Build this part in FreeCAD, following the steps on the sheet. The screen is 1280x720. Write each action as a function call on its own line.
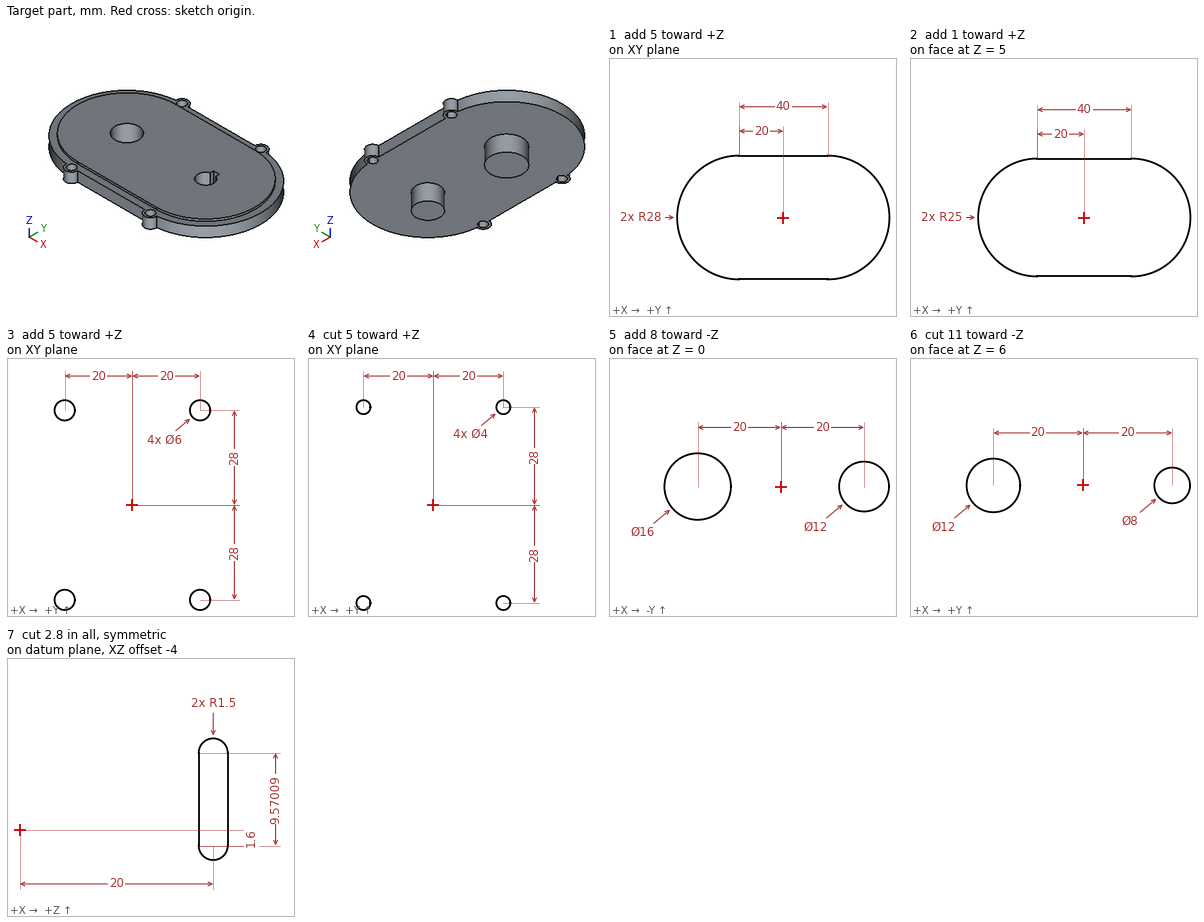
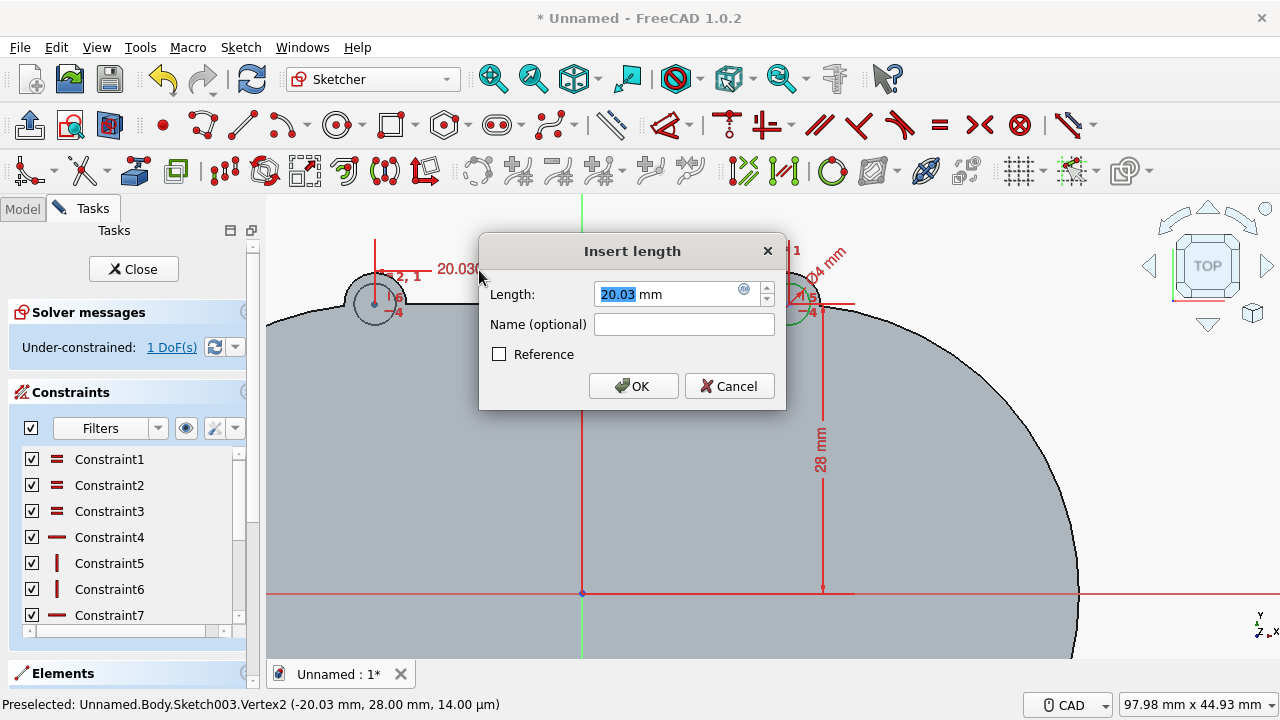
text(20)
key(Return)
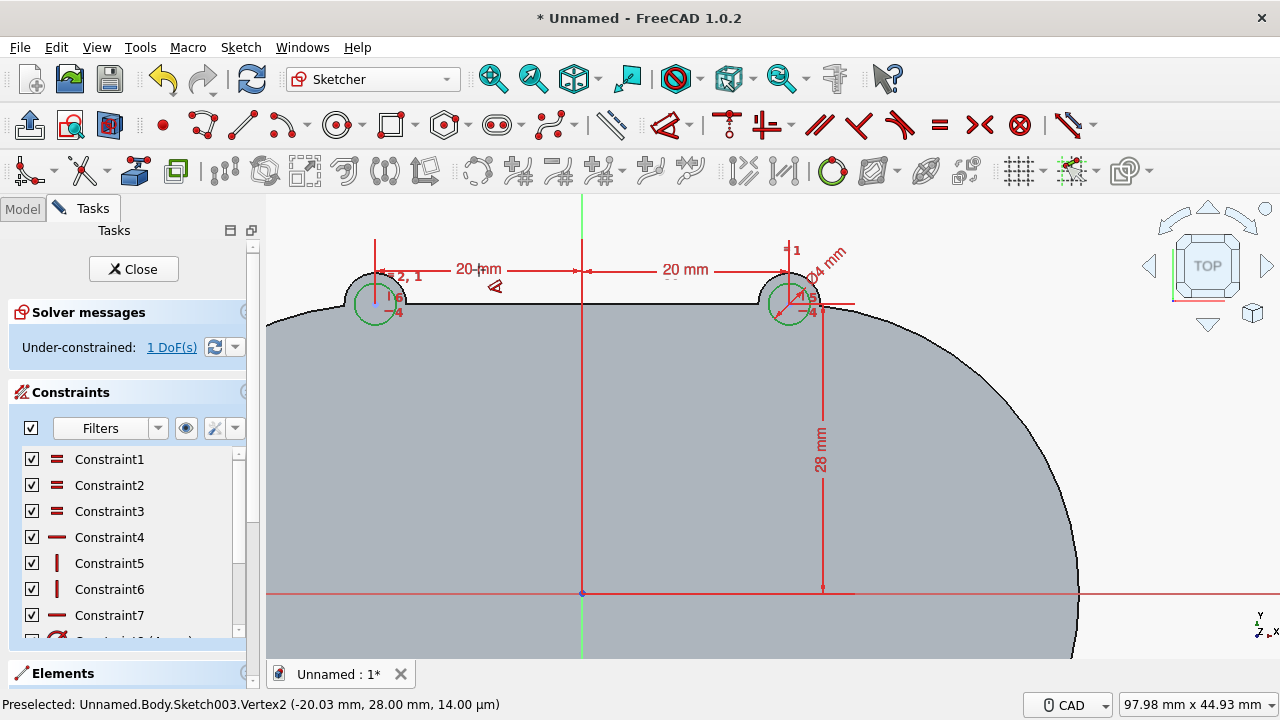
scroll(804, 290, down, 4)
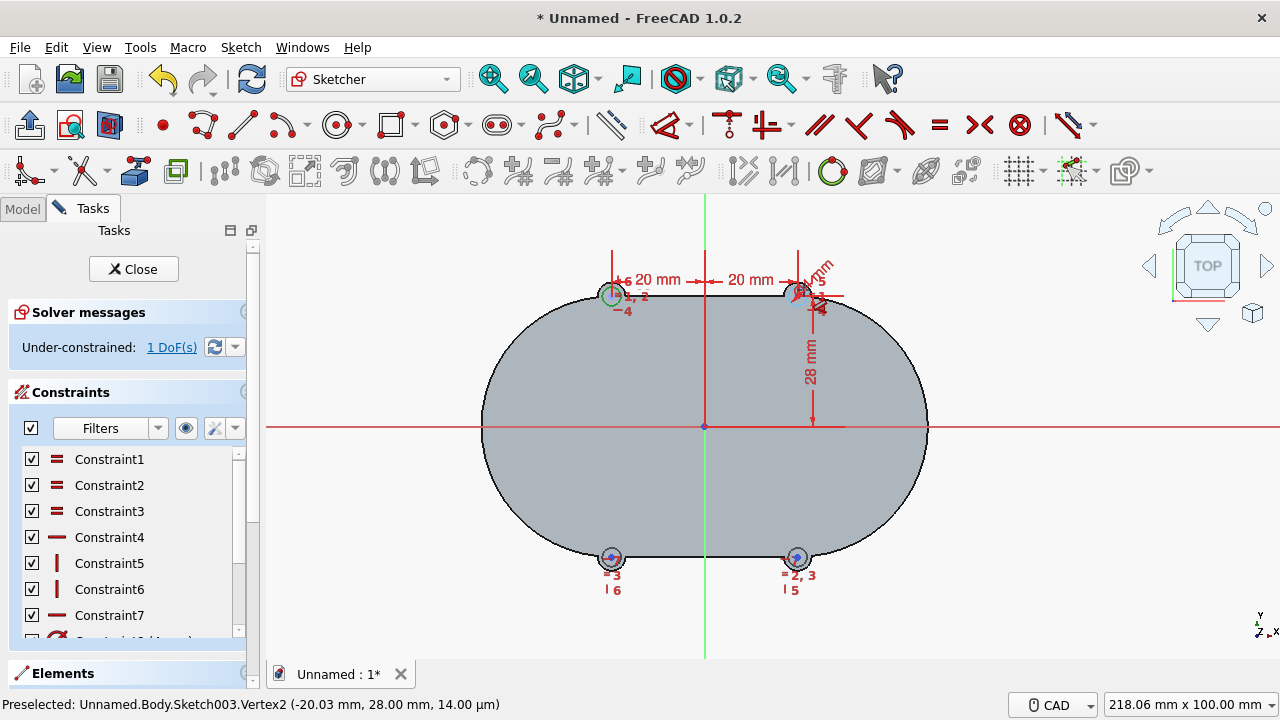
click(798, 557)
click(832, 492)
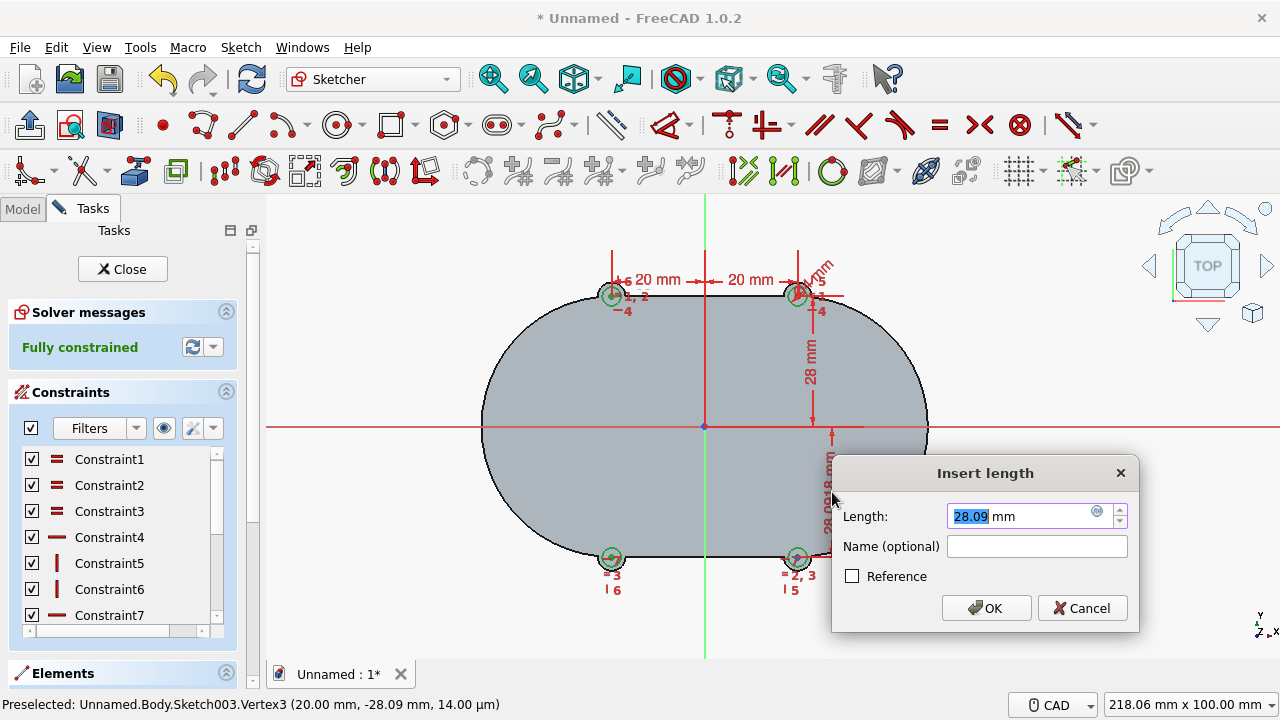
text(28)
key(Return)
key(Escape)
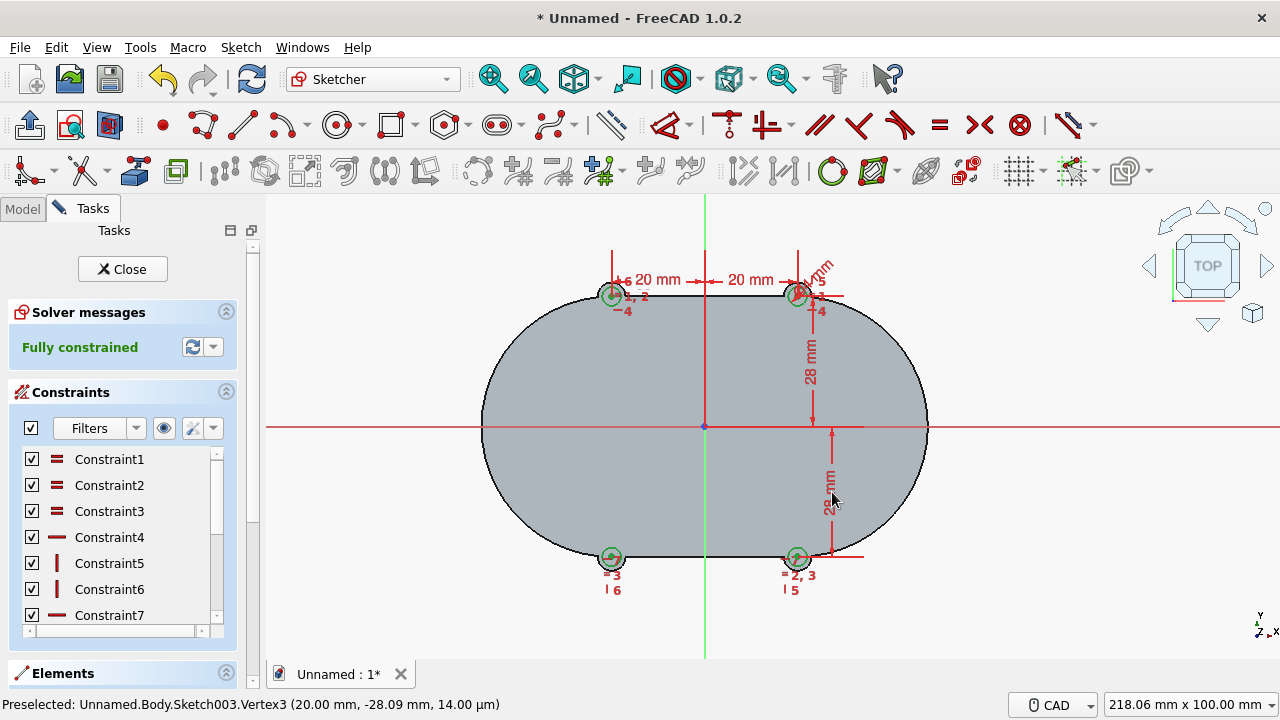
click(123, 269)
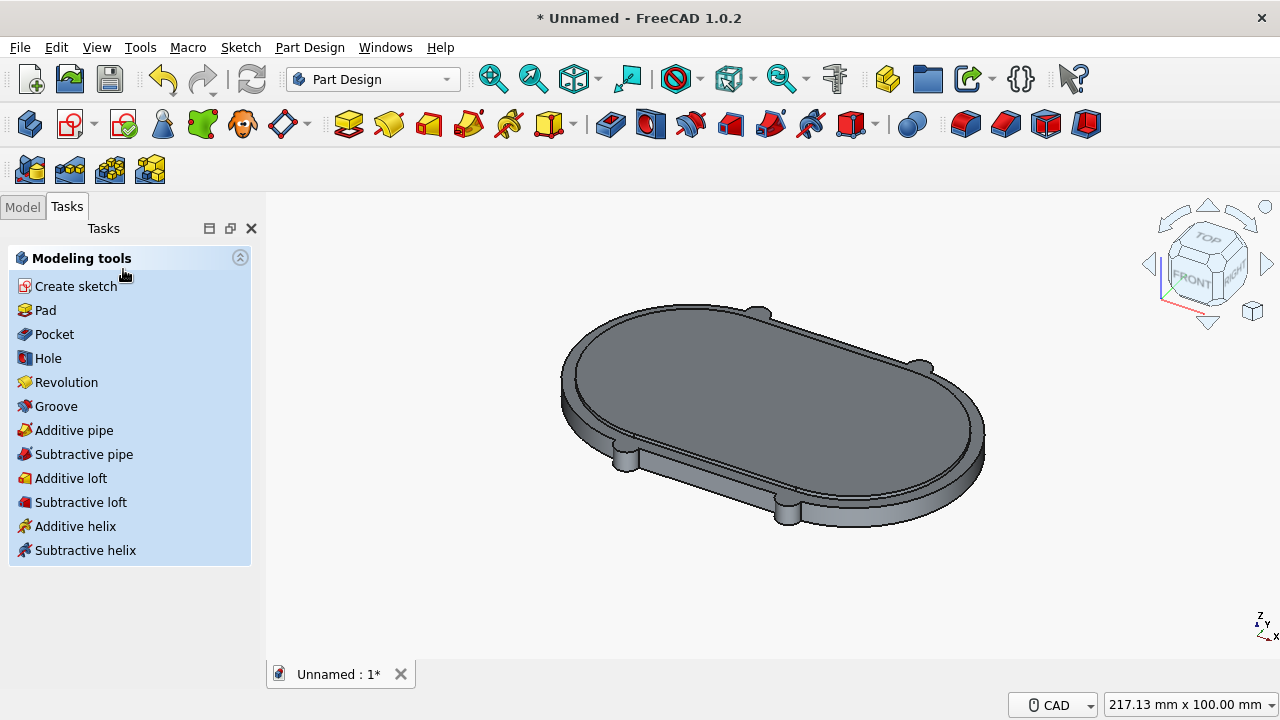
click(612, 124)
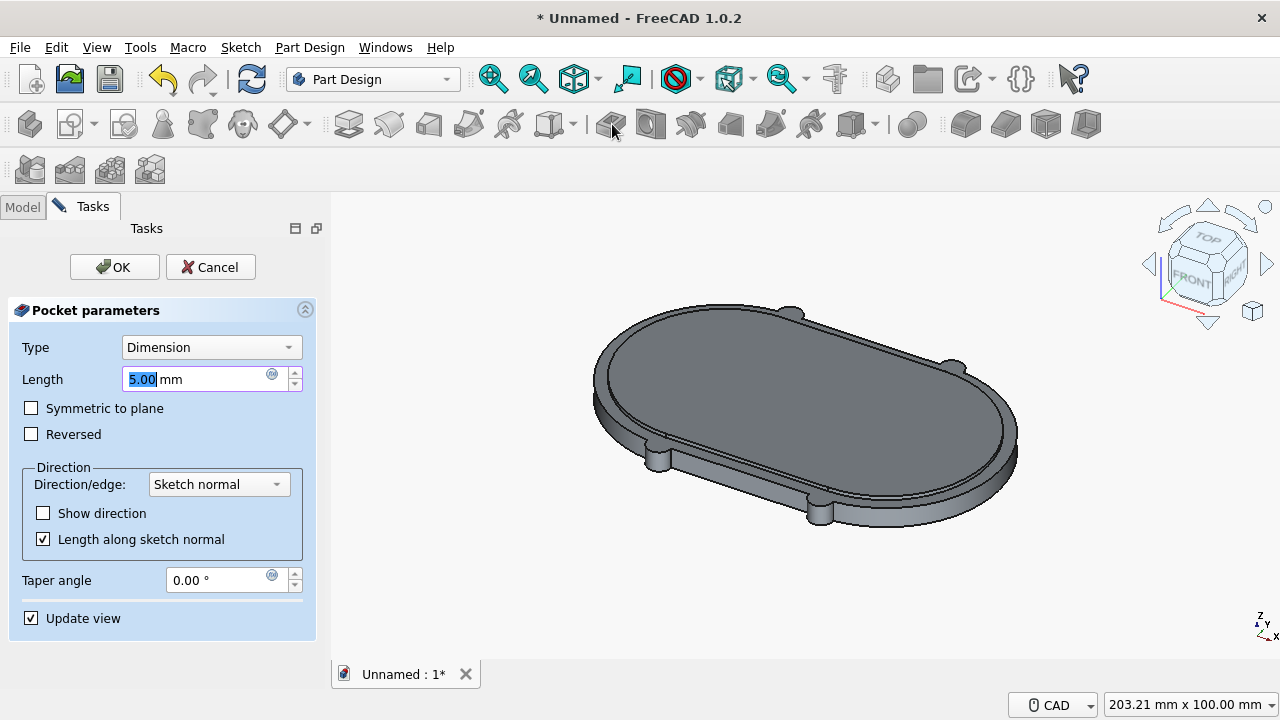
text(5)
key(Tab)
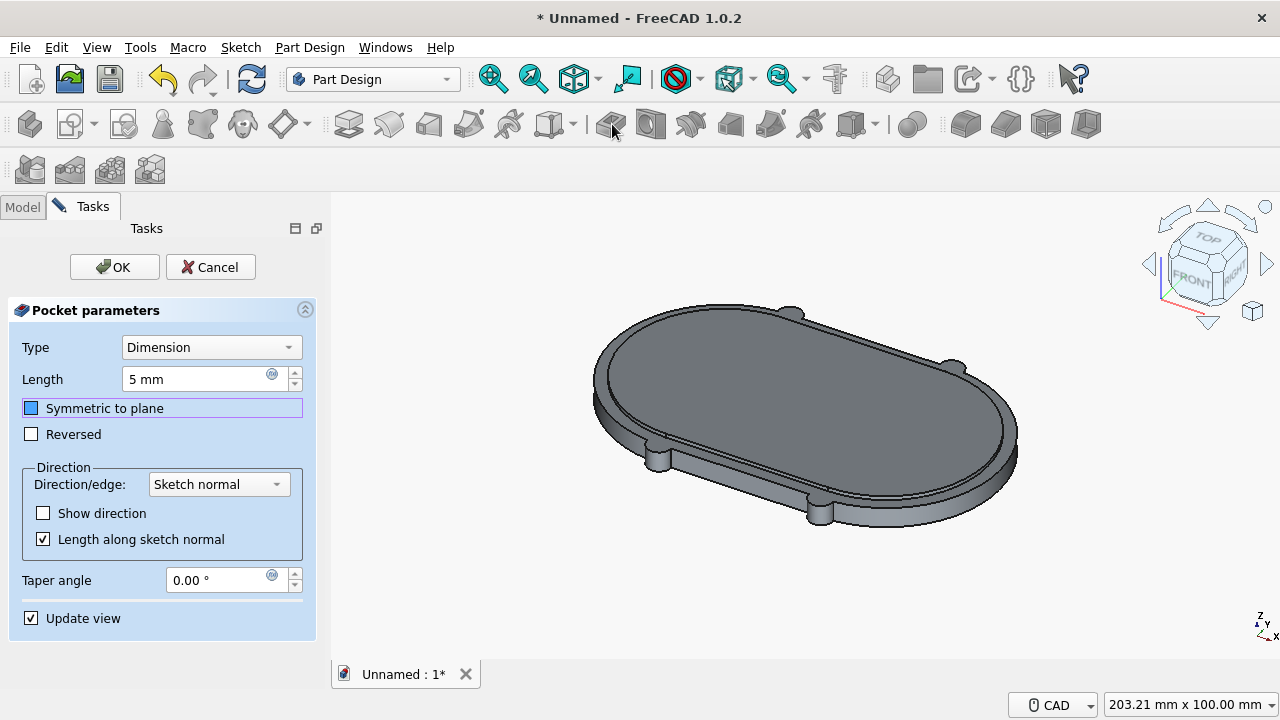
click(30, 434)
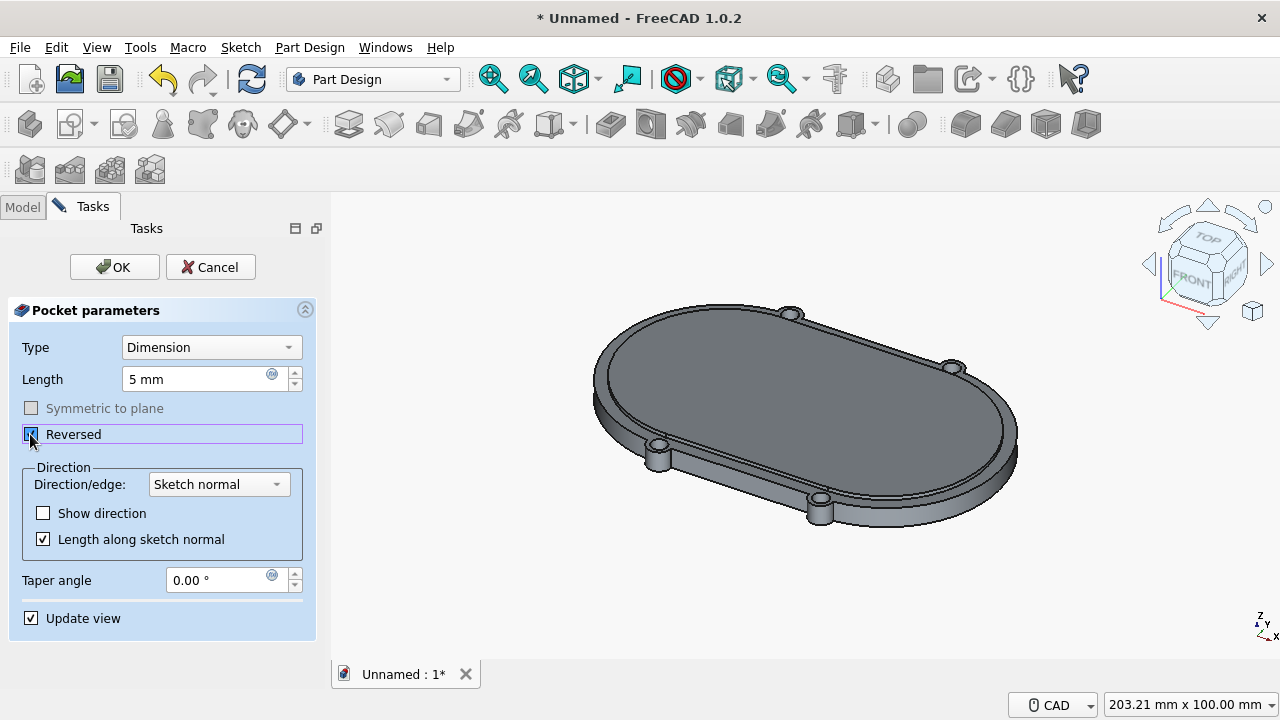
click(115, 267)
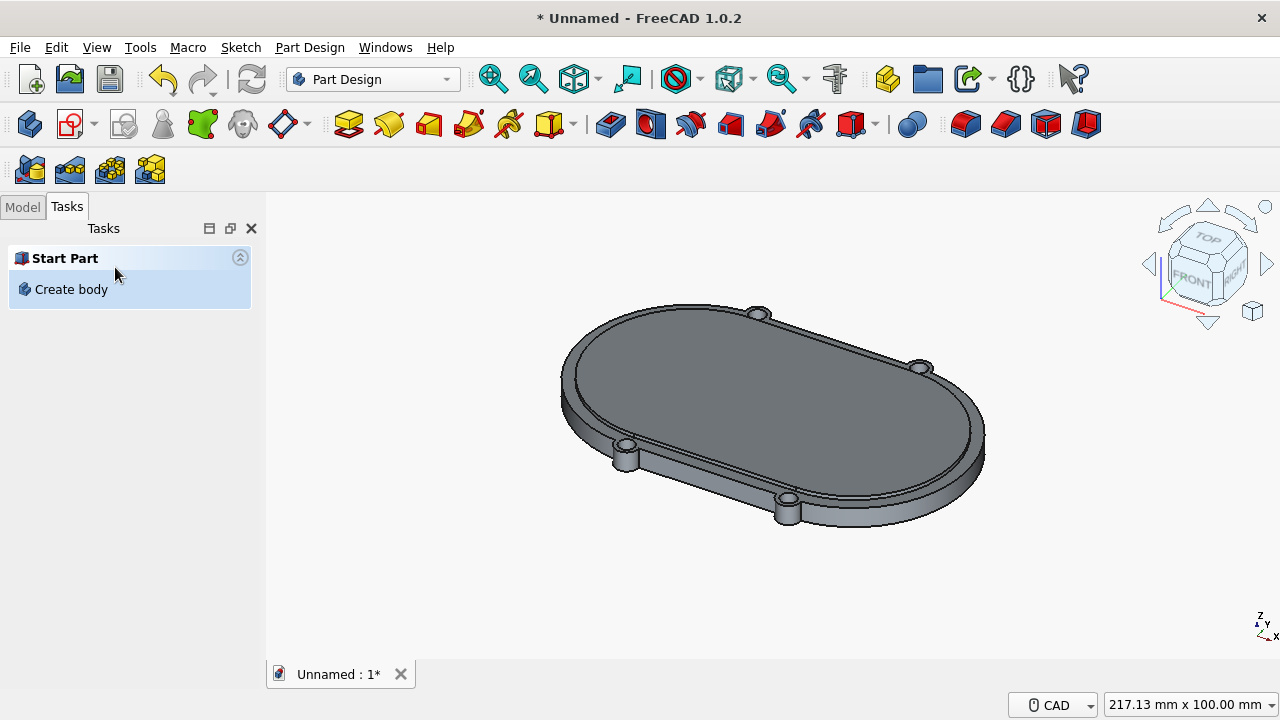
key(5)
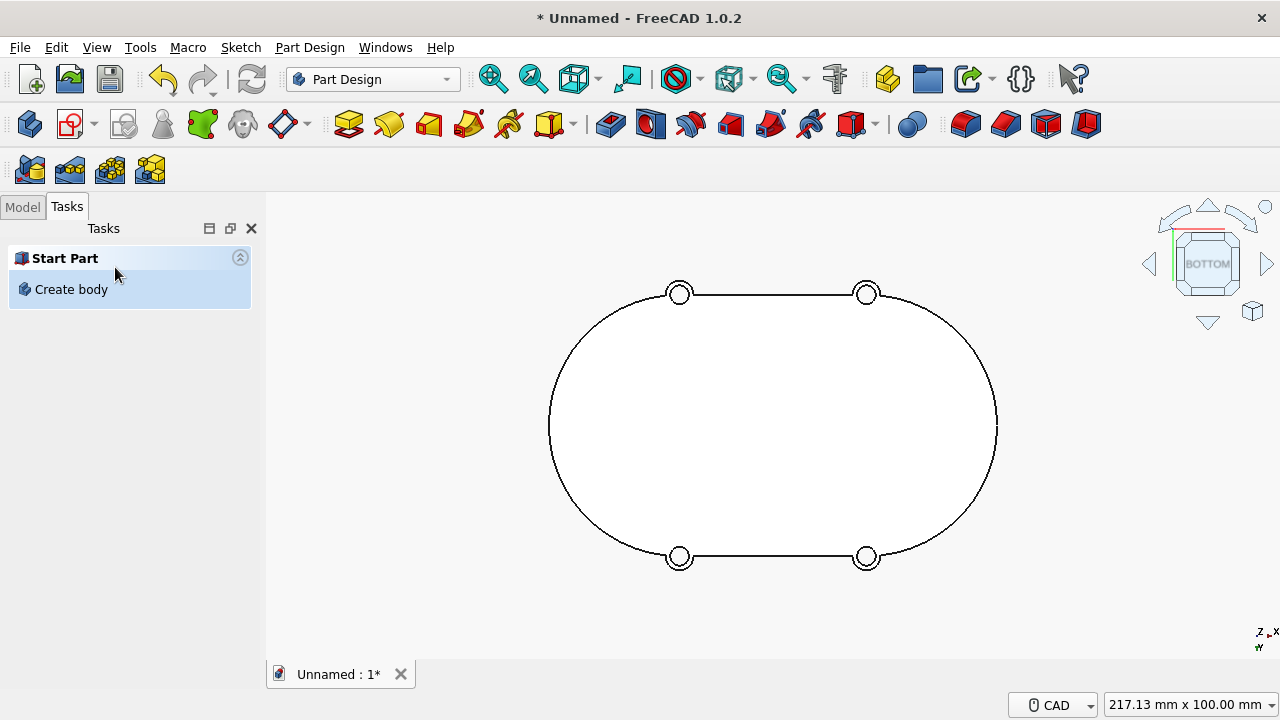
click(773, 424)